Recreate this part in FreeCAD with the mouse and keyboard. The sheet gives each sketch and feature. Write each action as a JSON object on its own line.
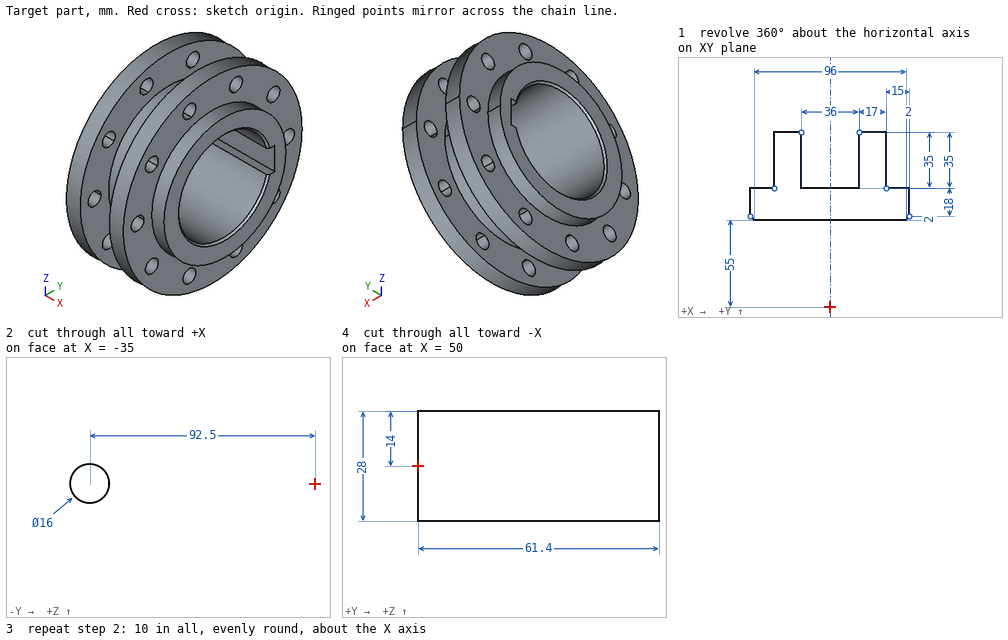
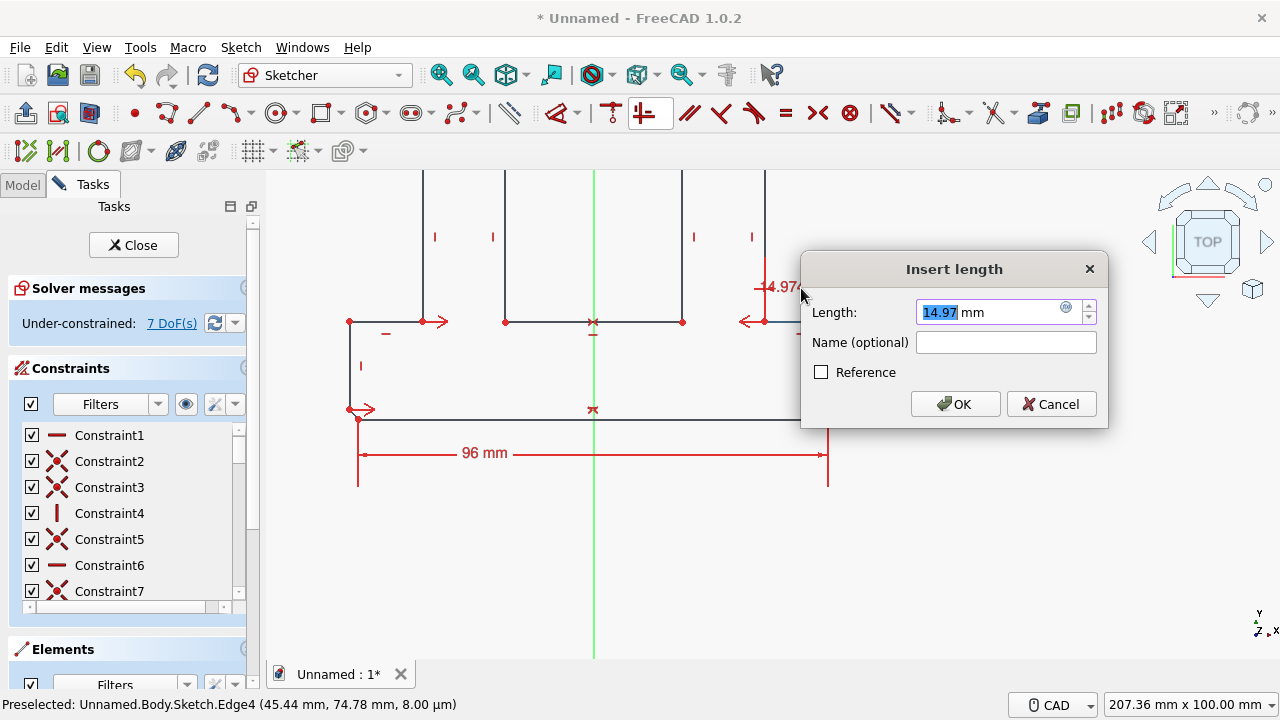
{"action": "type", "text": "15"}
{"action": "key", "text": "Return"}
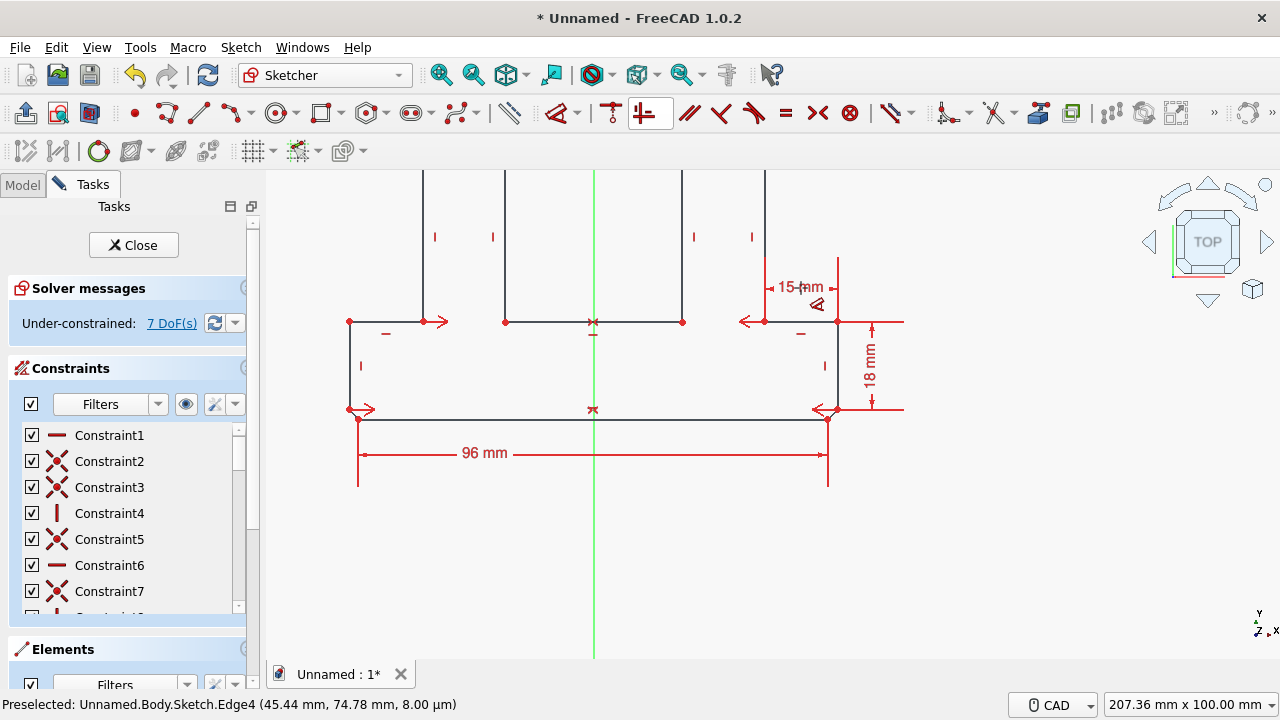
{"action": "left_click", "coordinate": [765, 270]}
{"action": "left_click", "coordinate": [799, 260]}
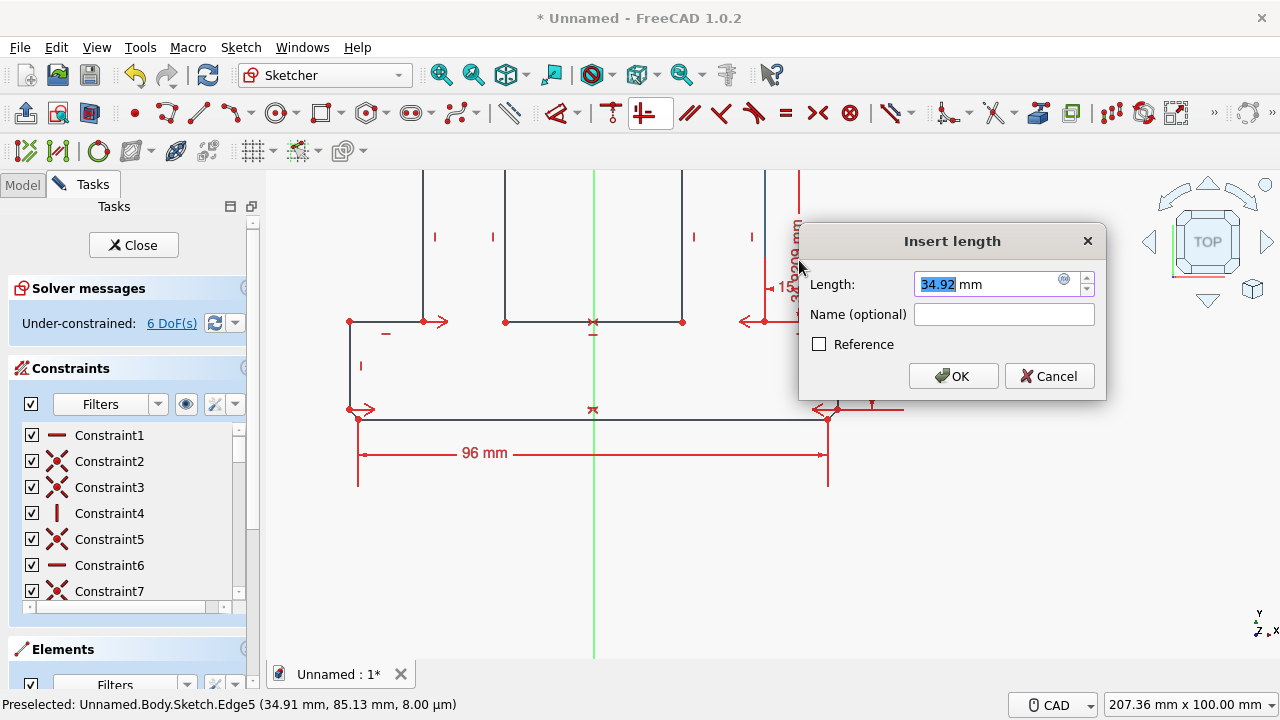
{"action": "type", "text": "35"}
{"action": "key", "text": "Return"}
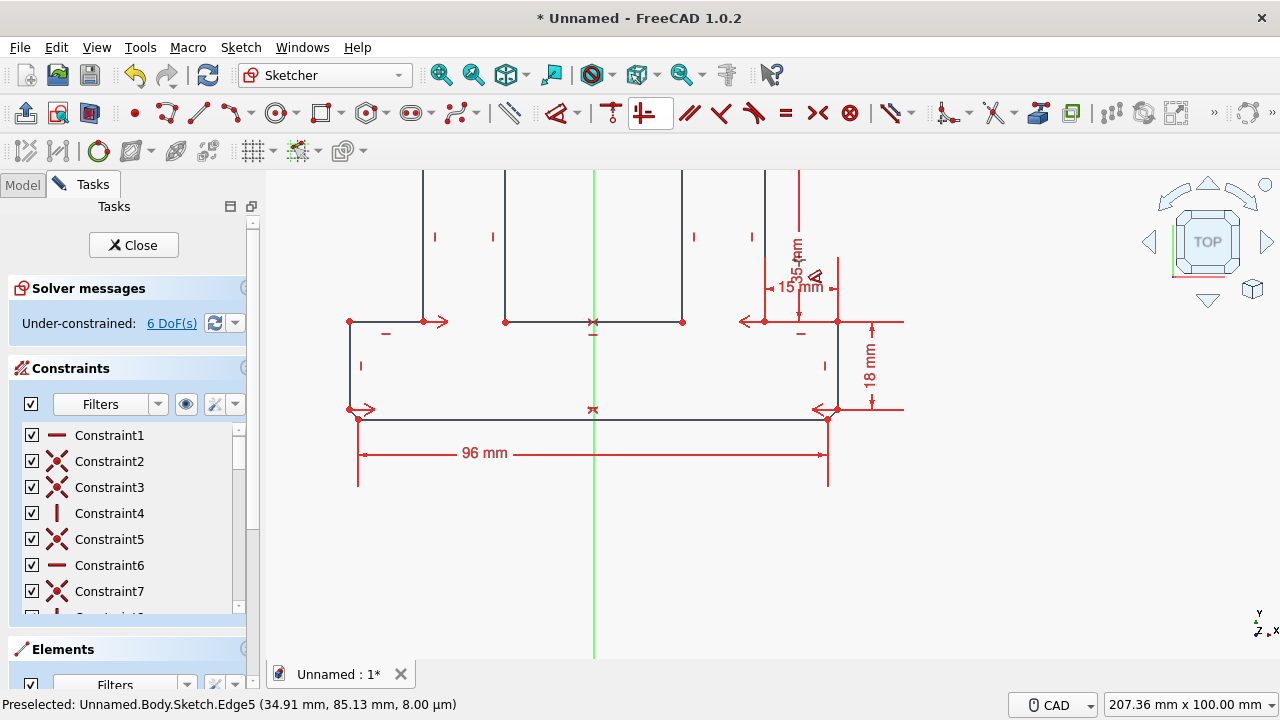
{"action": "scroll", "coordinate": [839, 410], "scroll_direction": "down", "scroll_amount": 3}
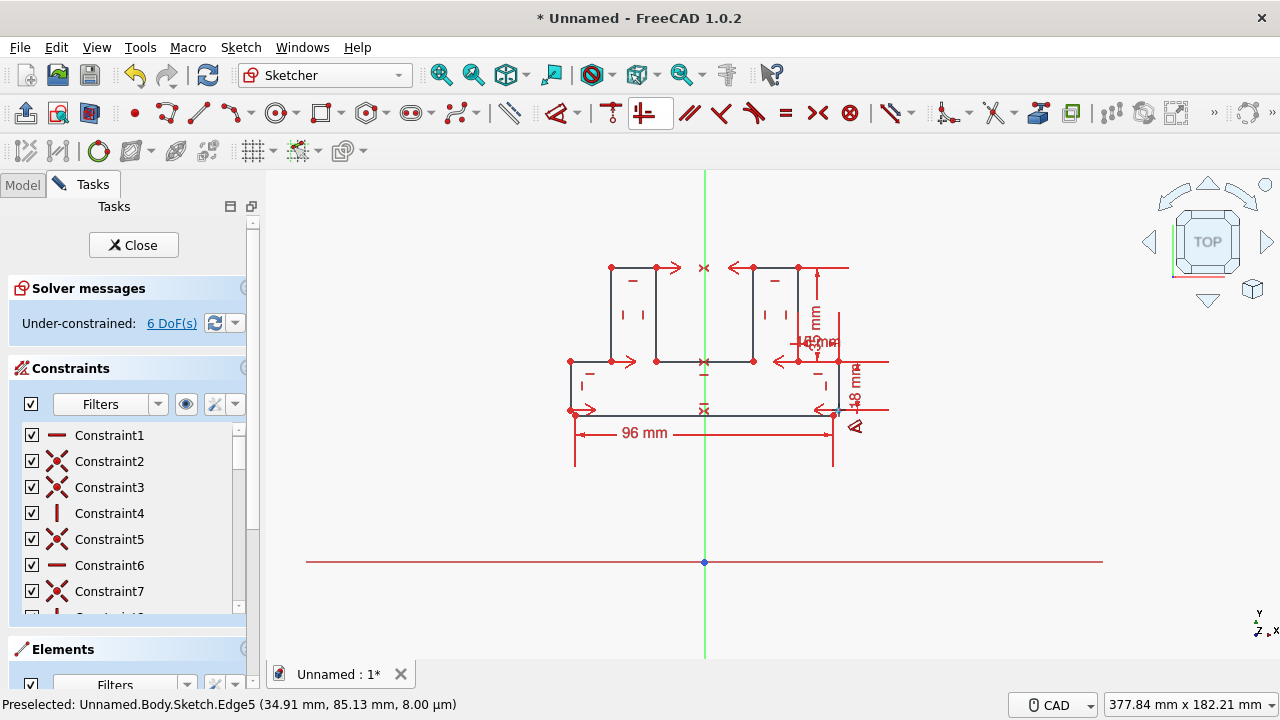
{"action": "left_click", "coordinate": [785, 268]}
{"action": "left_click", "coordinate": [776, 234]}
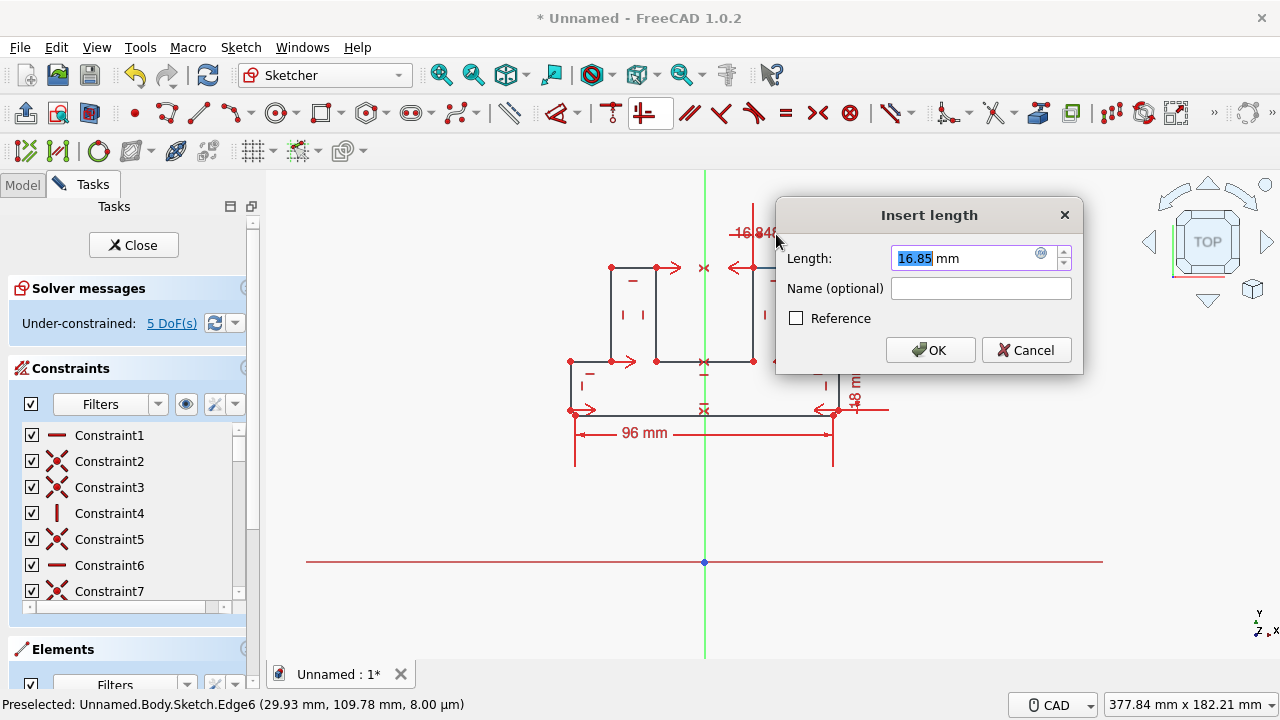
{"action": "type", "text": "17"}
{"action": "key", "text": "Return"}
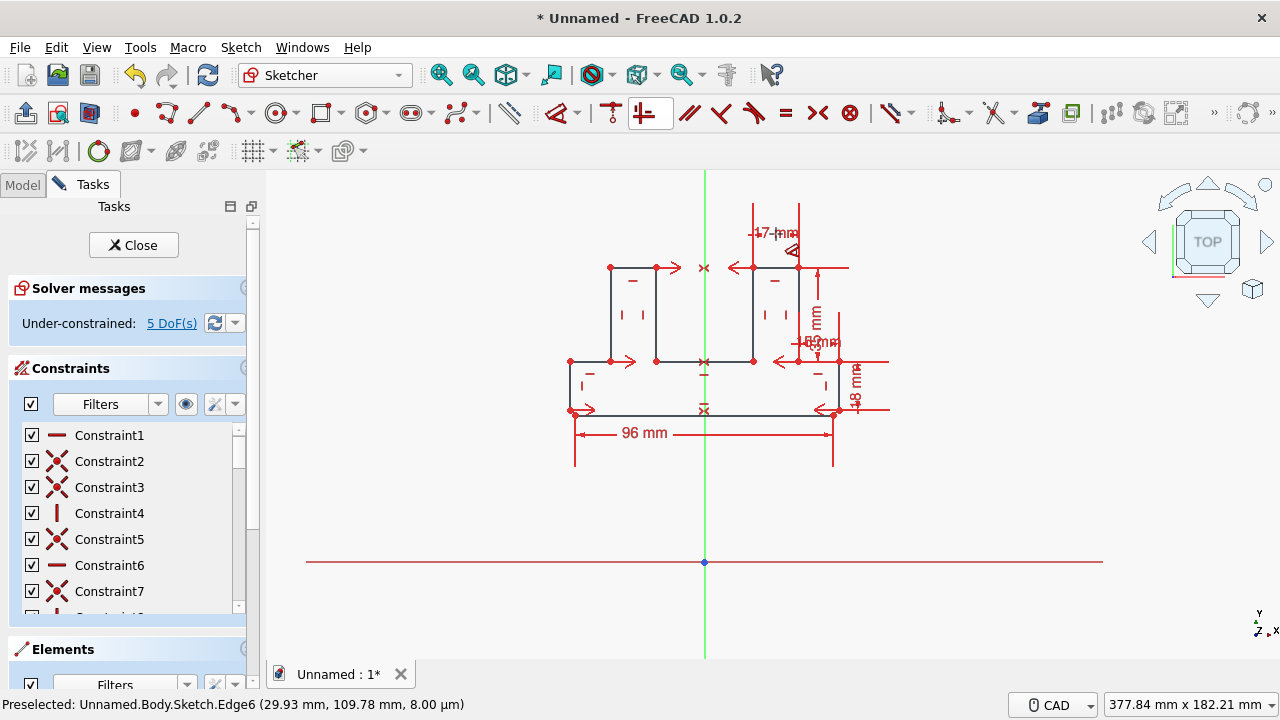
{"action": "left_click", "coordinate": [753, 296]}
{"action": "left_click", "coordinate": [719, 315]}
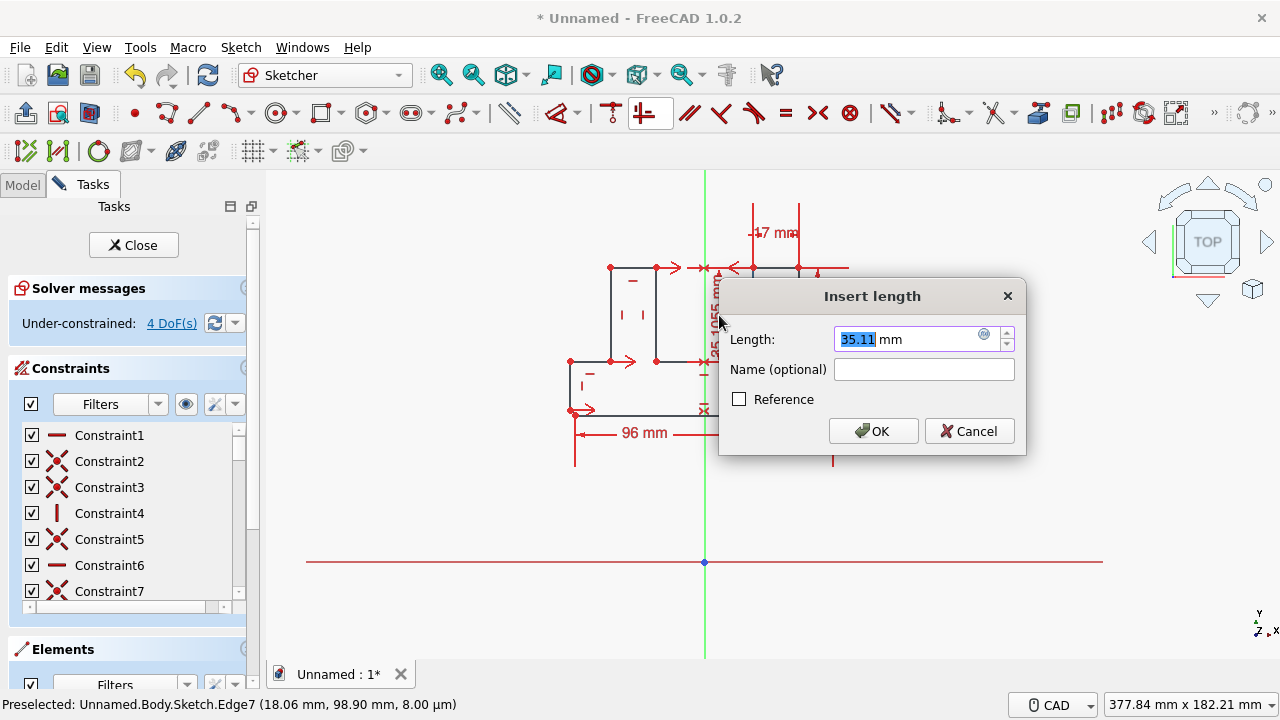
{"action": "type", "text": "35"}
{"action": "key", "text": "Return"}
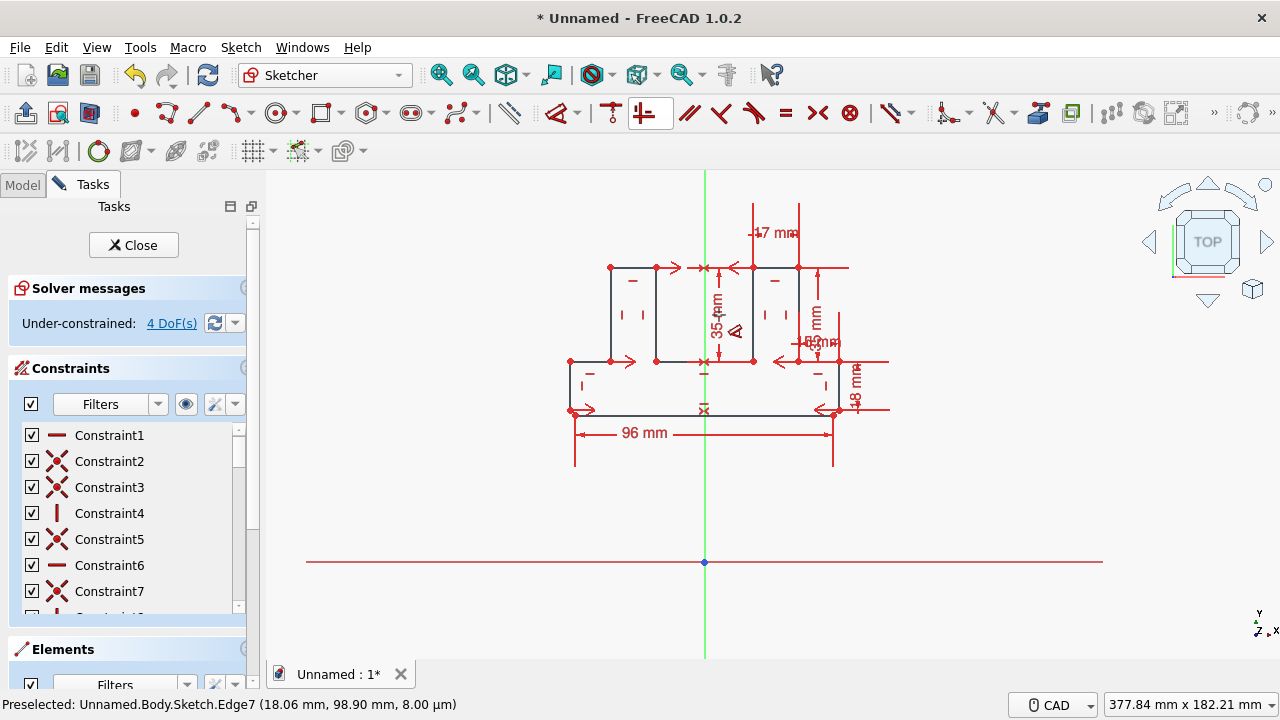
{"action": "left_click", "coordinate": [724, 362]}
{"action": "left_click", "coordinate": [682, 396]}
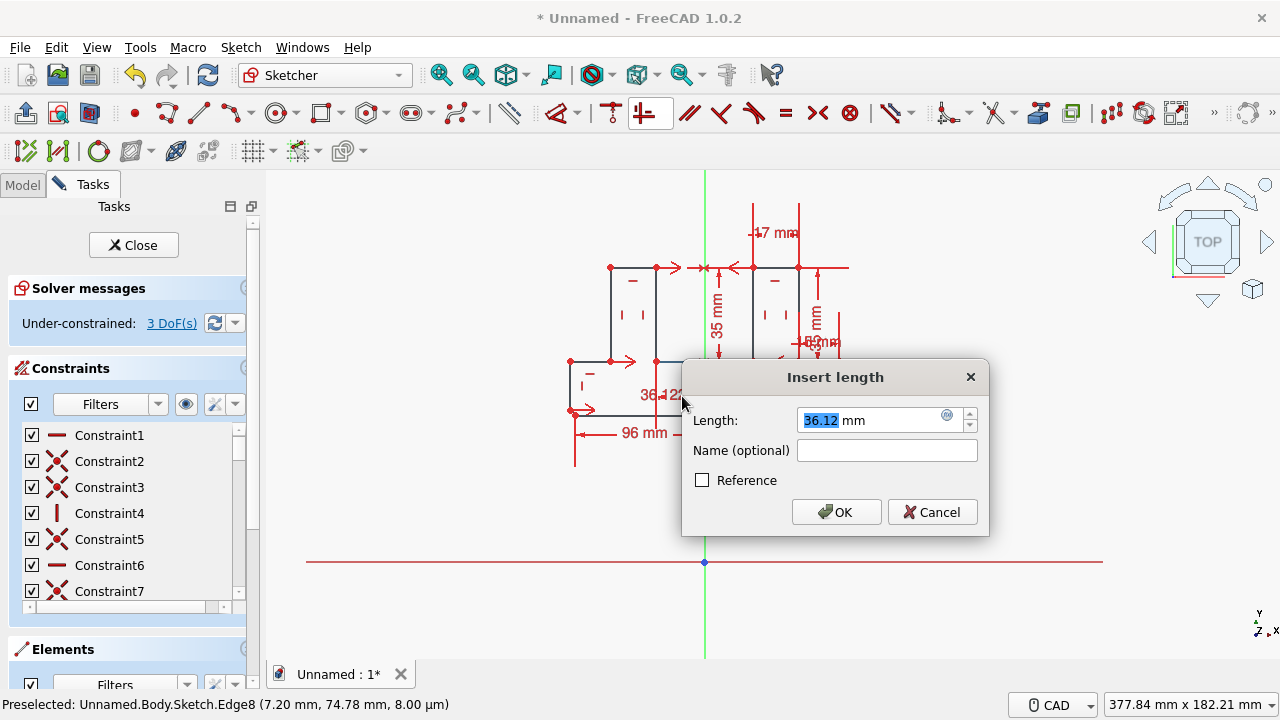
{"action": "type", "text": "36"}
{"action": "key", "text": "Return"}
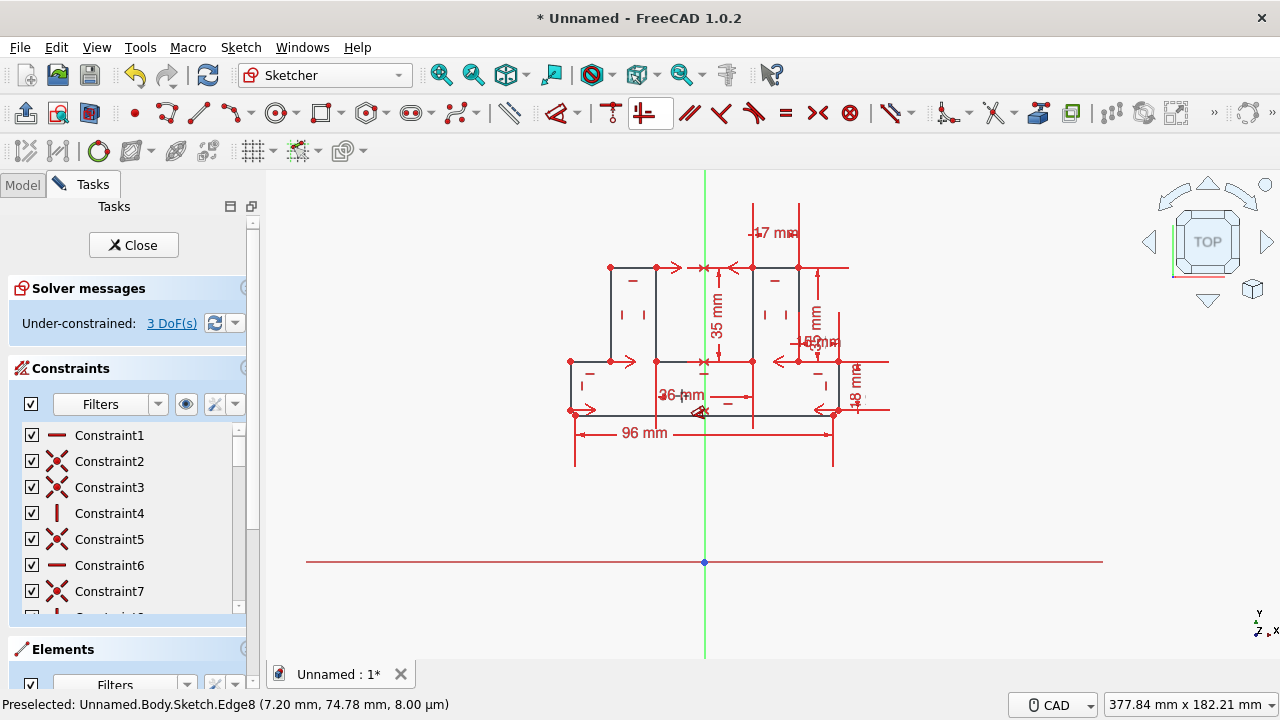
{"action": "scroll", "coordinate": [836, 413], "scroll_direction": "up", "scroll_amount": 11}